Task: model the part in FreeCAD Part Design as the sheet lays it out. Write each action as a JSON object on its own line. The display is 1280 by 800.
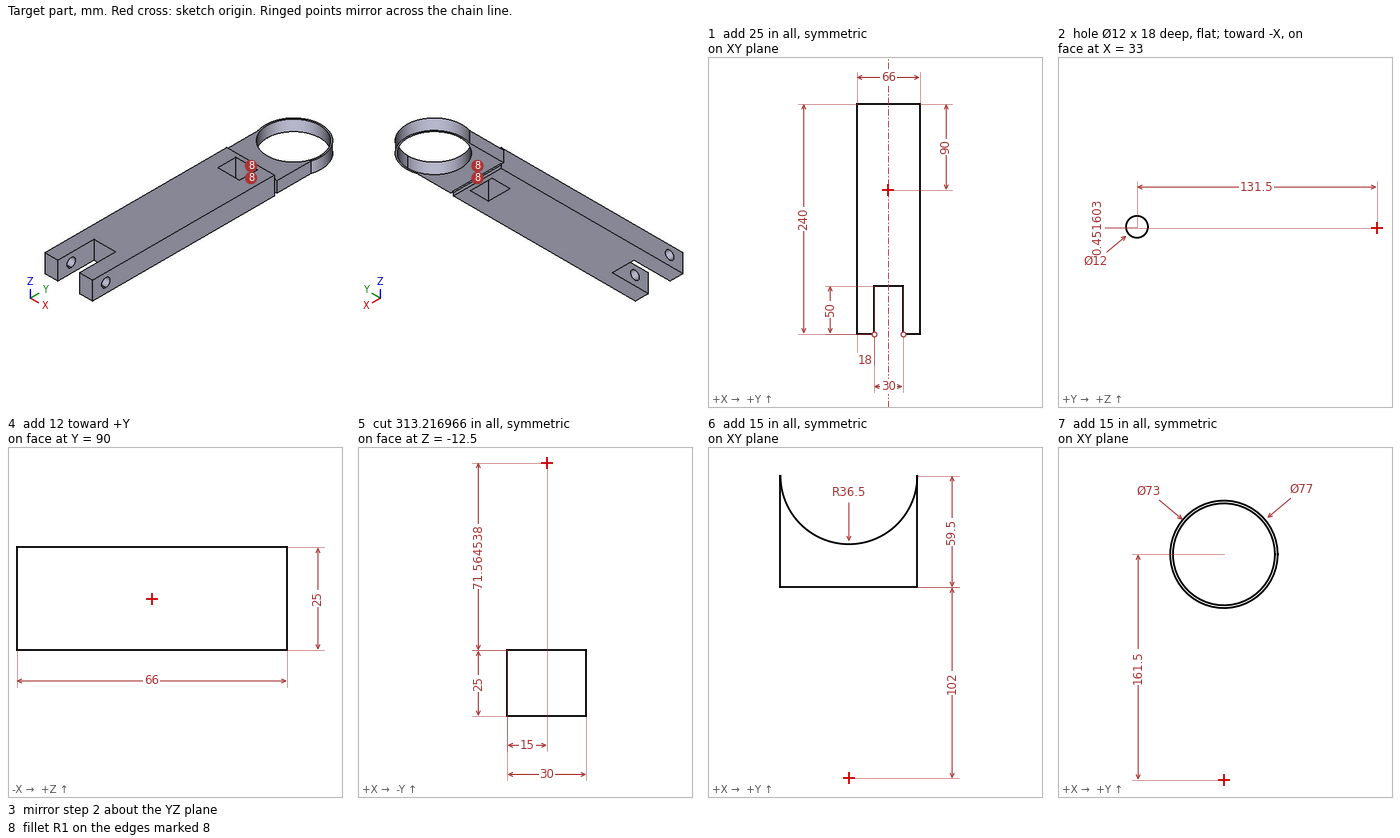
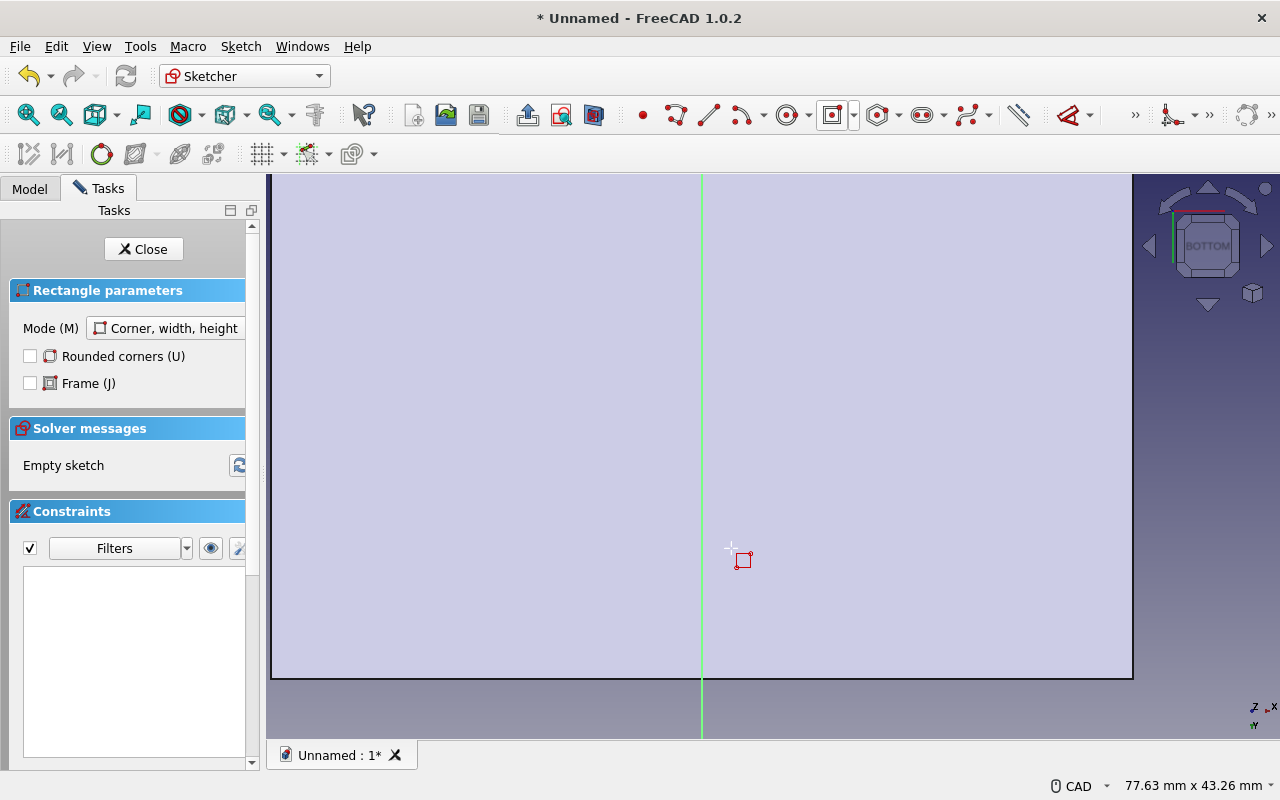
{"action": "left_click", "coordinate": [506, 281]}
{"action": "left_click", "coordinate": [898, 608]}
{"action": "key", "text": "Escape"}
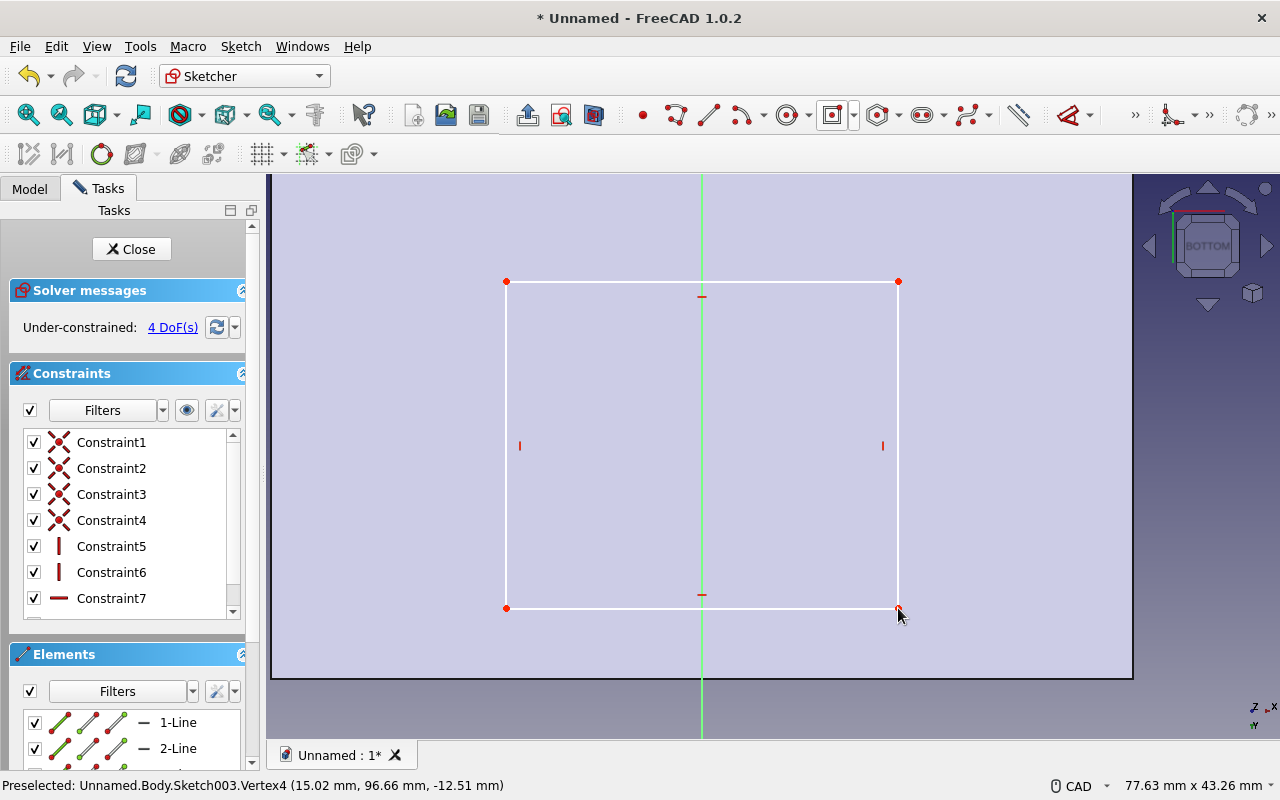
{"action": "left_click", "coordinate": [1068, 116]}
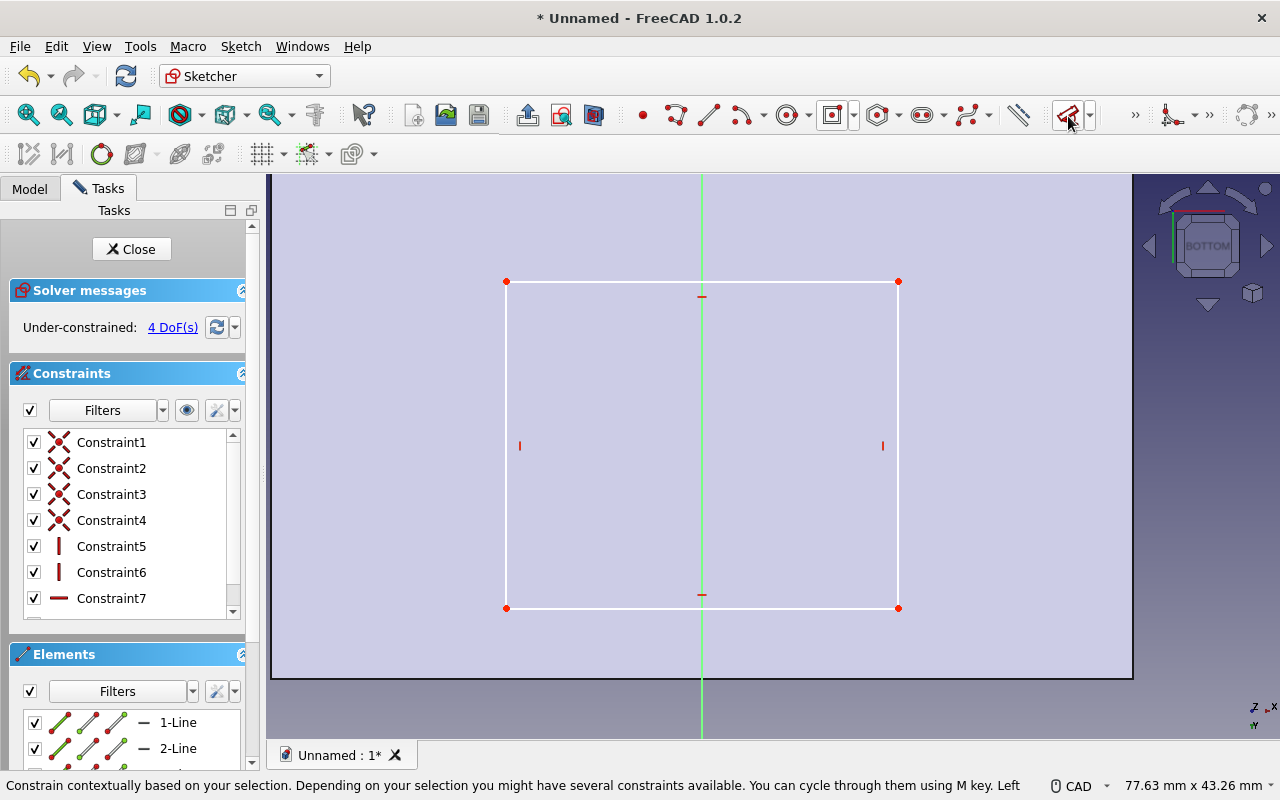
{"action": "left_click", "coordinate": [506, 380]}
{"action": "left_click", "coordinate": [472, 446]}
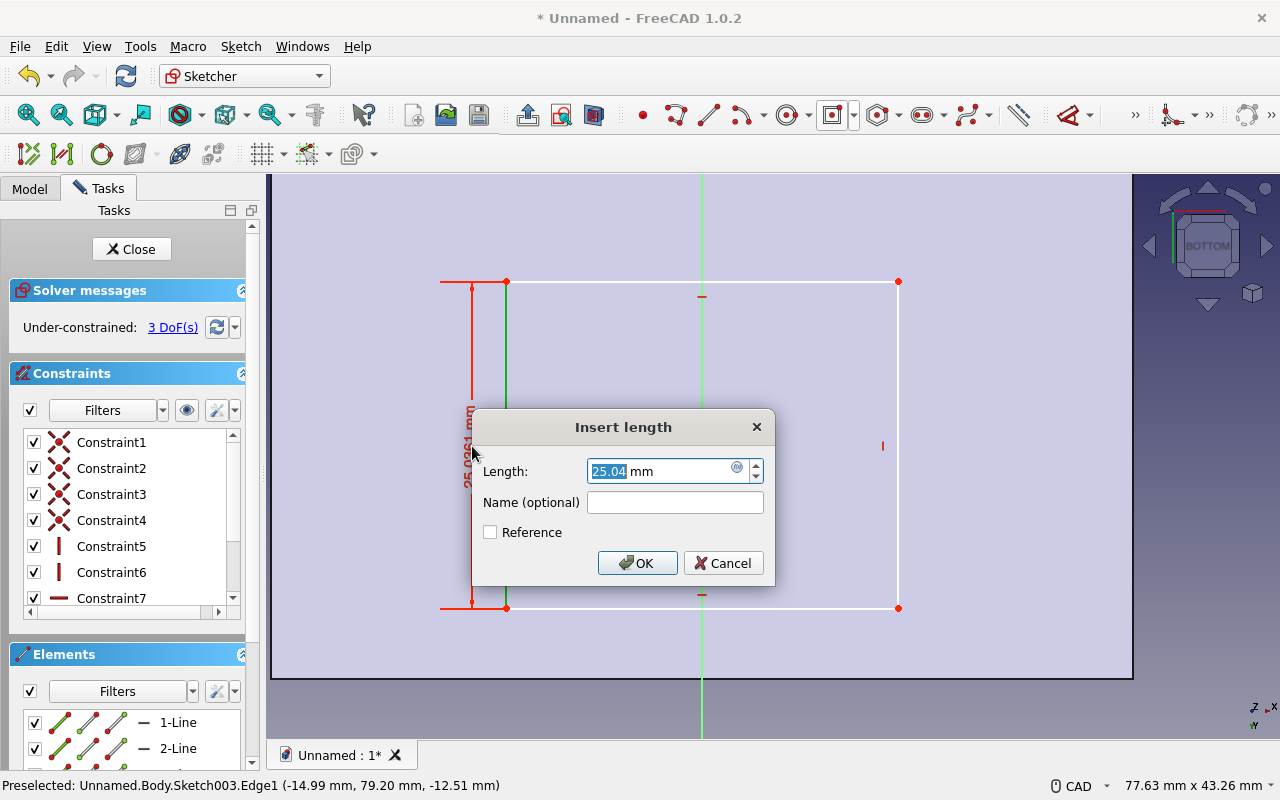
{"action": "type", "text": "25"}
{"action": "key", "text": "Return"}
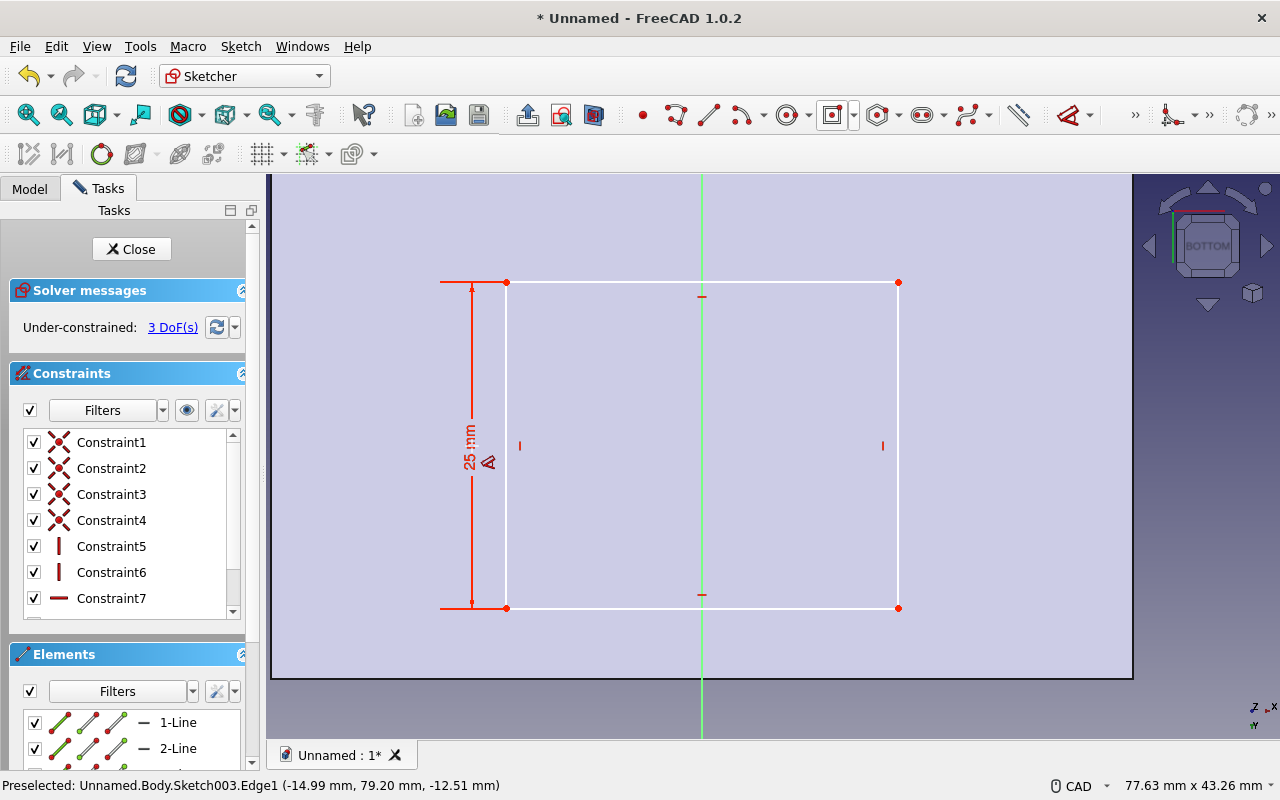
{"action": "left_click", "coordinate": [624, 609]}
{"action": "left_click", "coordinate": [612, 643]}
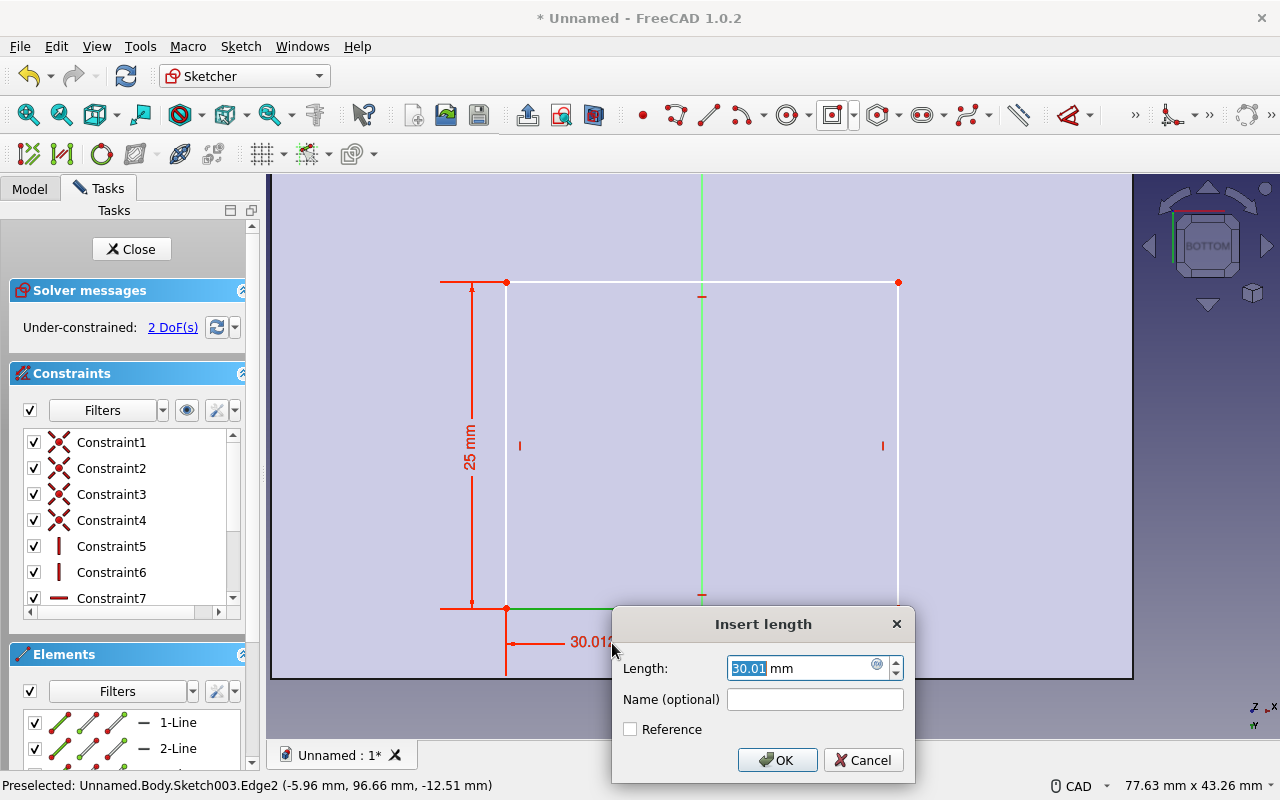
{"action": "type", "text": "30"}
{"action": "key", "text": "Return"}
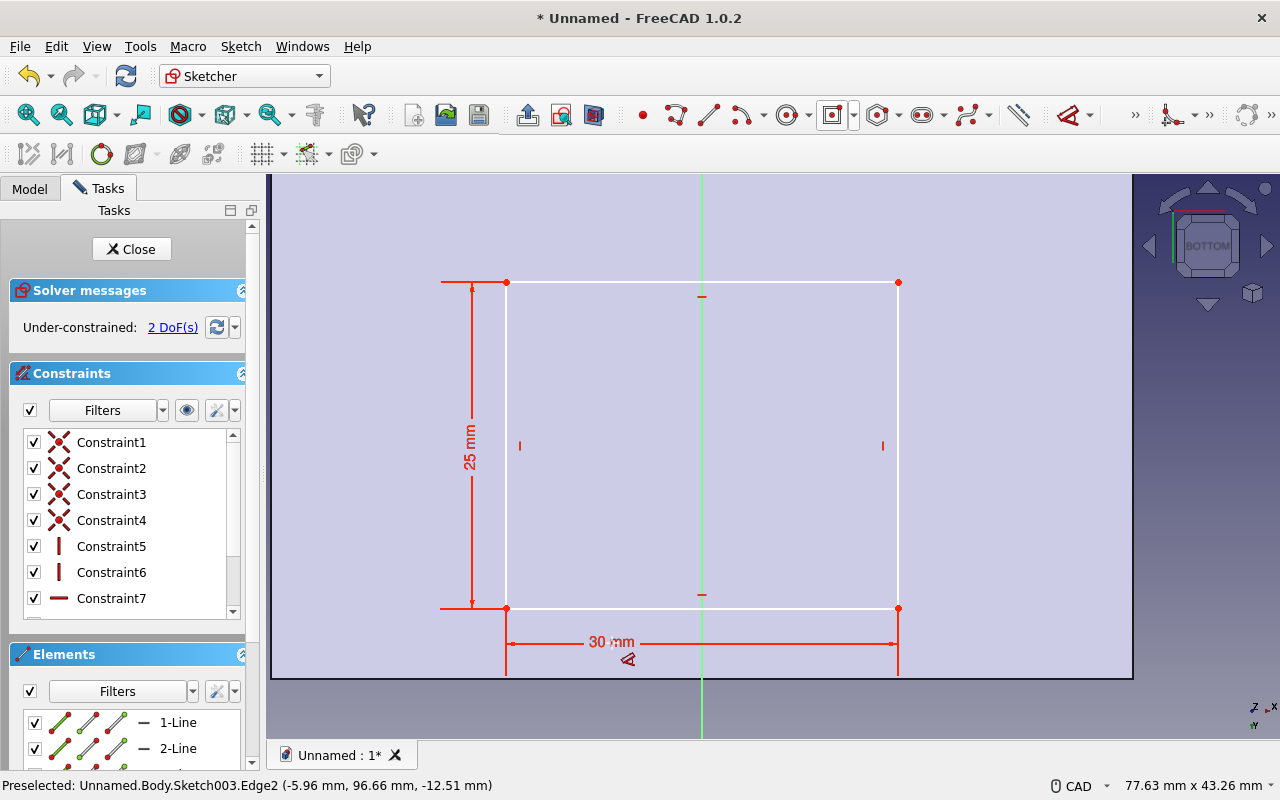
{"action": "left_click", "coordinate": [506, 282]}
{"action": "left_click", "coordinate": [604, 316]}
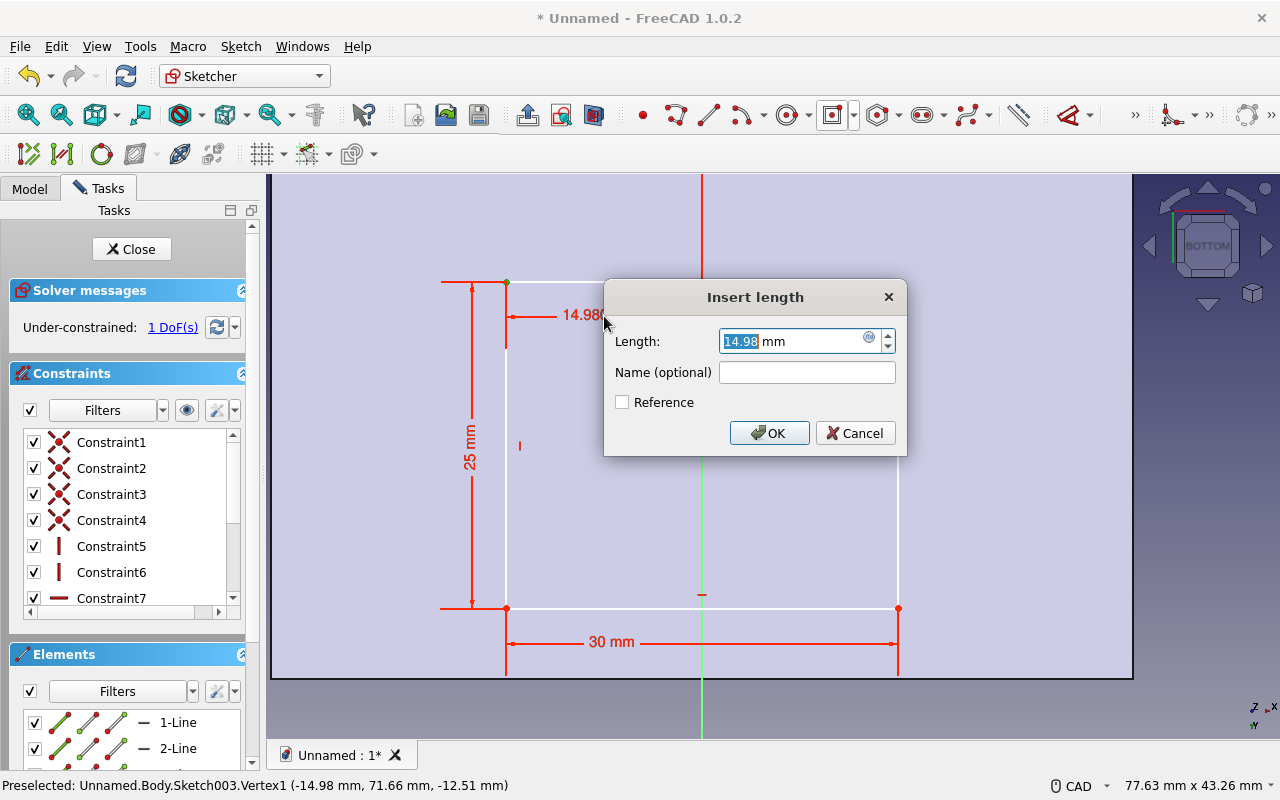
{"action": "type", "text": "15"}
{"action": "key", "text": "Return"}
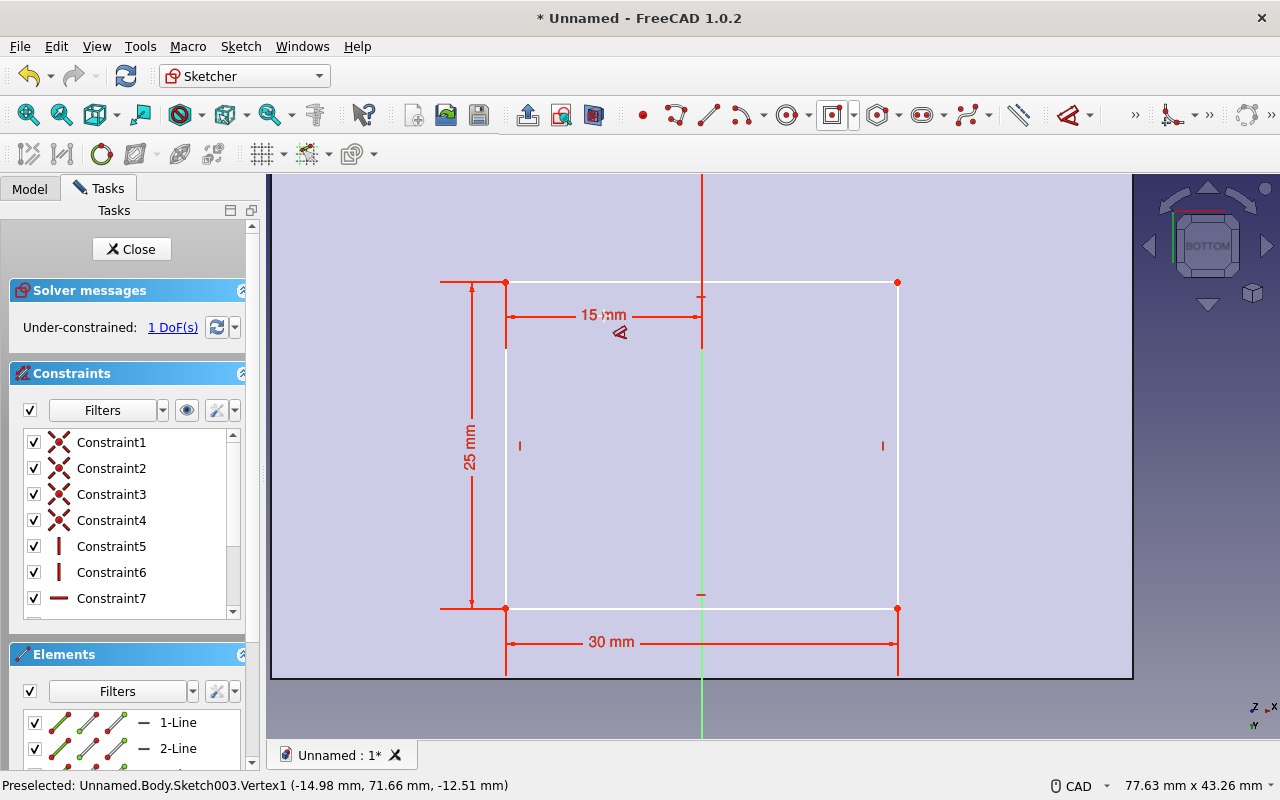
{"action": "left_click", "coordinate": [506, 282]}
{"action": "left_click", "coordinate": [472, 242]}